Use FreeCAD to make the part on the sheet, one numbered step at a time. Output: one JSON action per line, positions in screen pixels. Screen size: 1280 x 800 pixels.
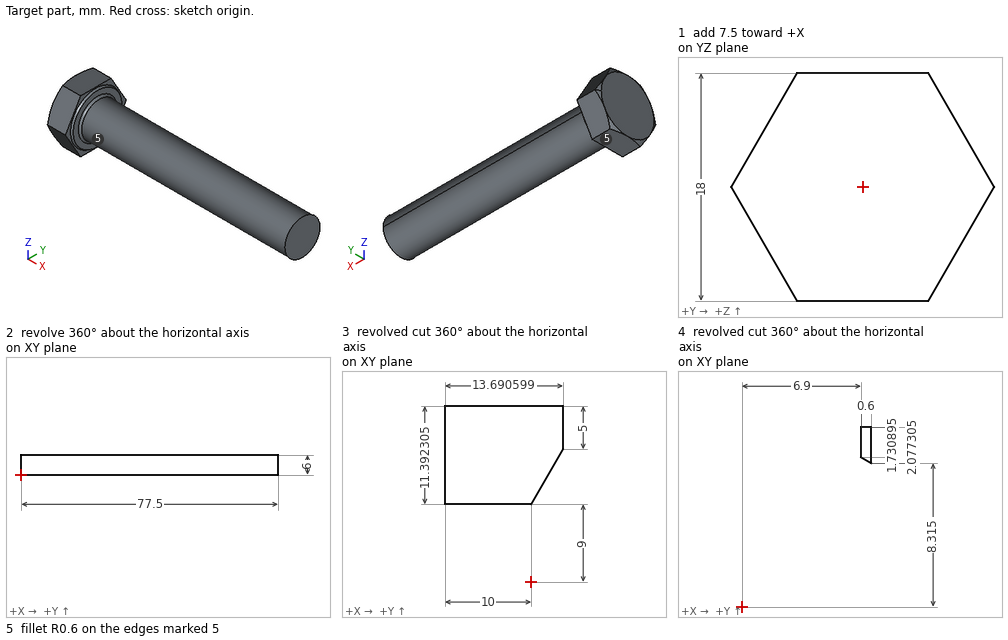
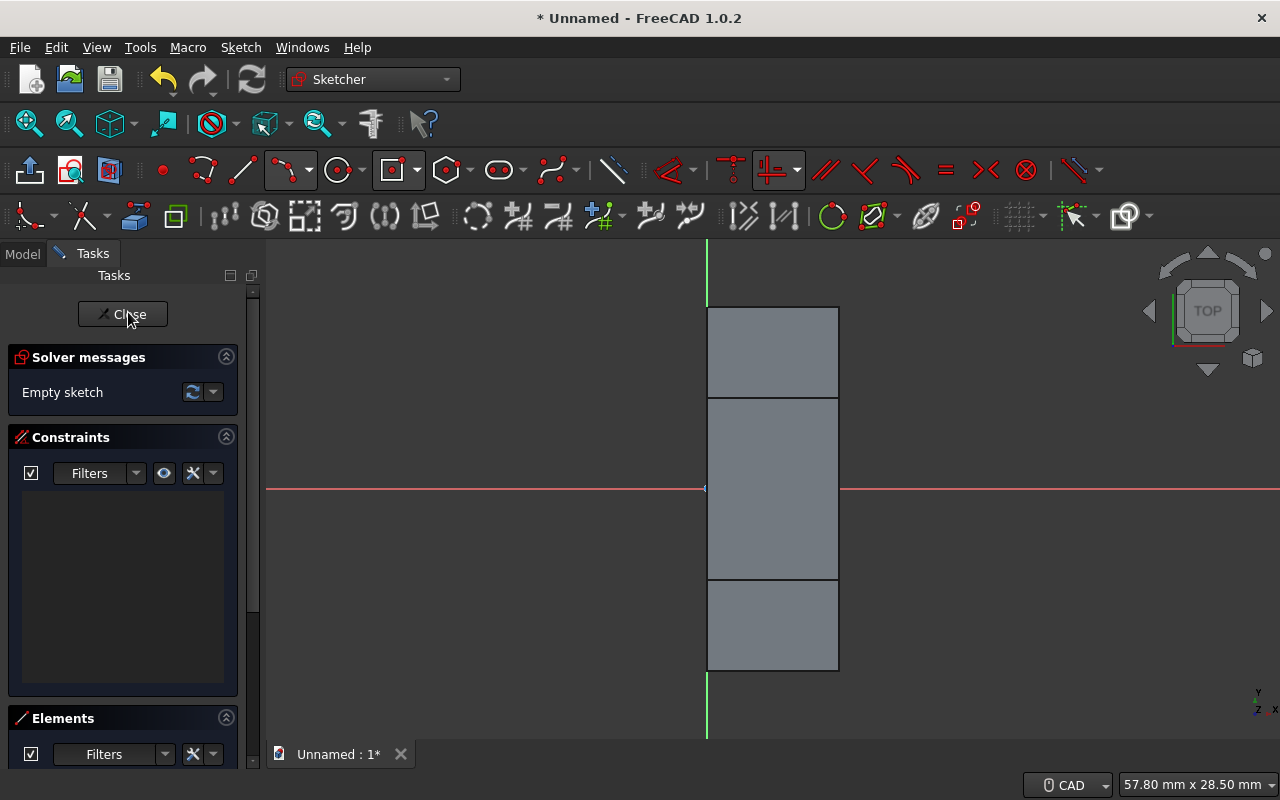
{"action": "left_click", "coordinate": [110, 170]}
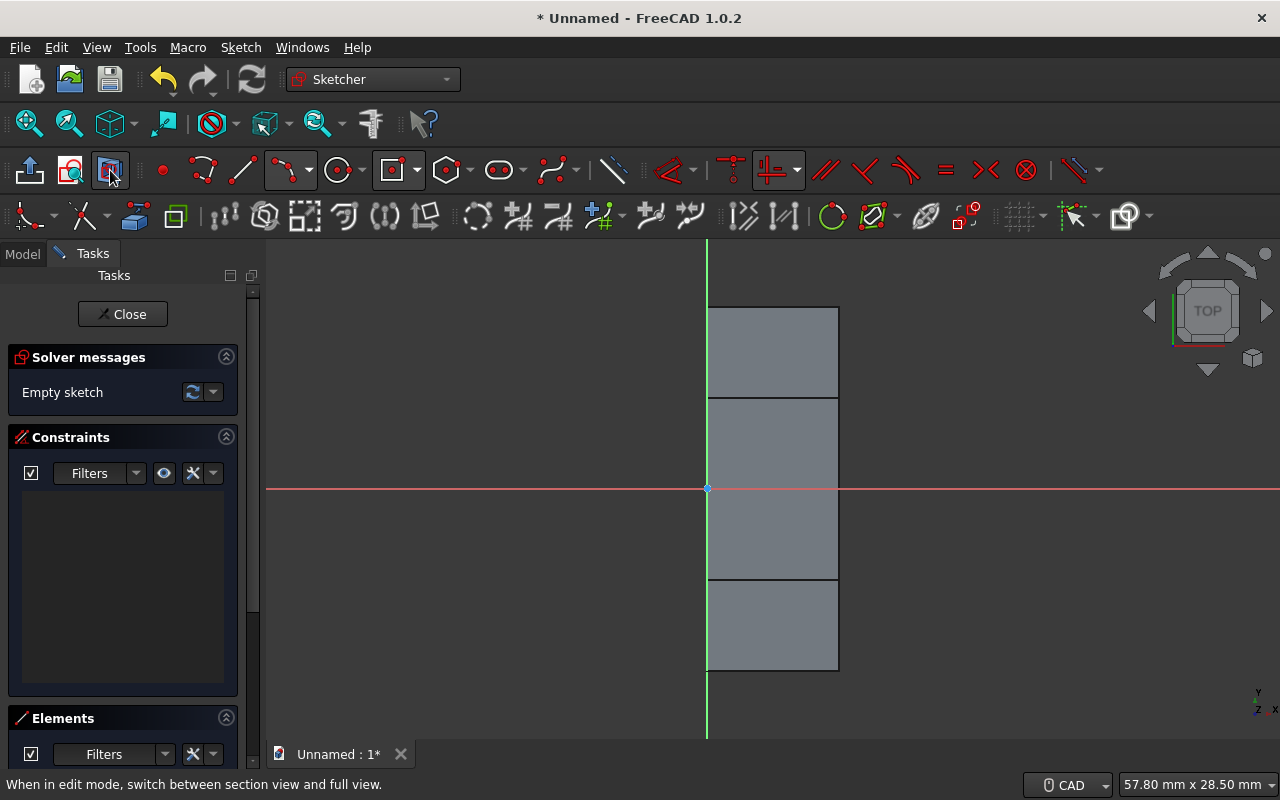
{"action": "scroll", "coordinate": [307, 520], "scroll_direction": "down", "scroll_amount": 5}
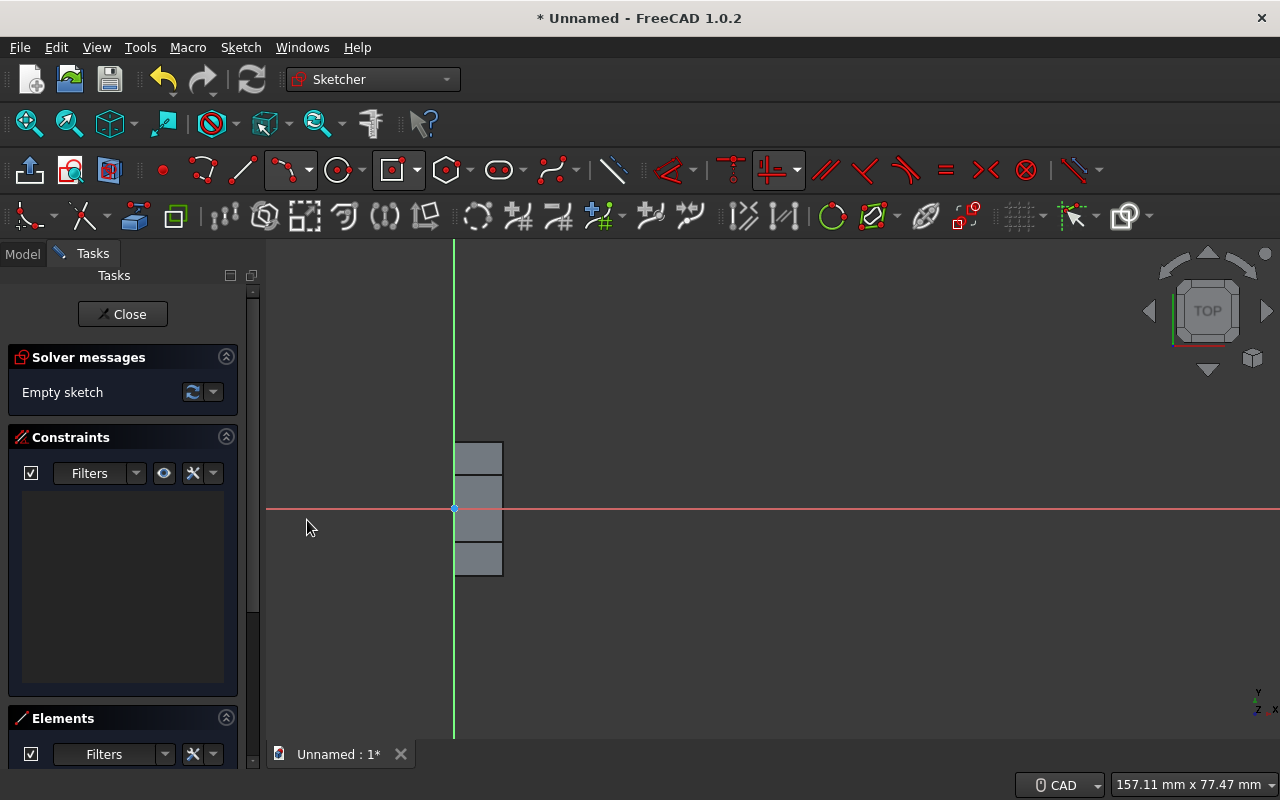
{"action": "key", "text": "g r"}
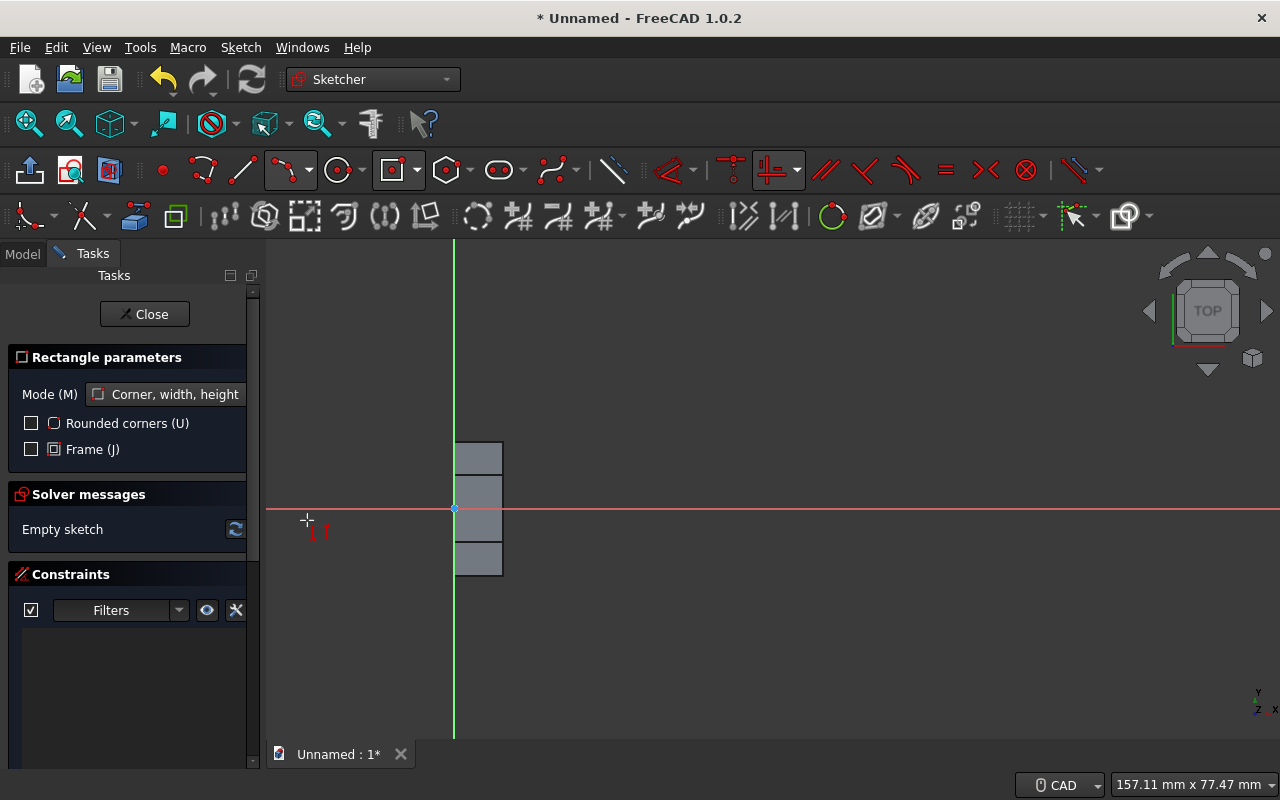
{"action": "left_click", "coordinate": [454, 509]}
{"action": "left_click", "coordinate": [954, 470]}
{"action": "key", "text": "Escape"}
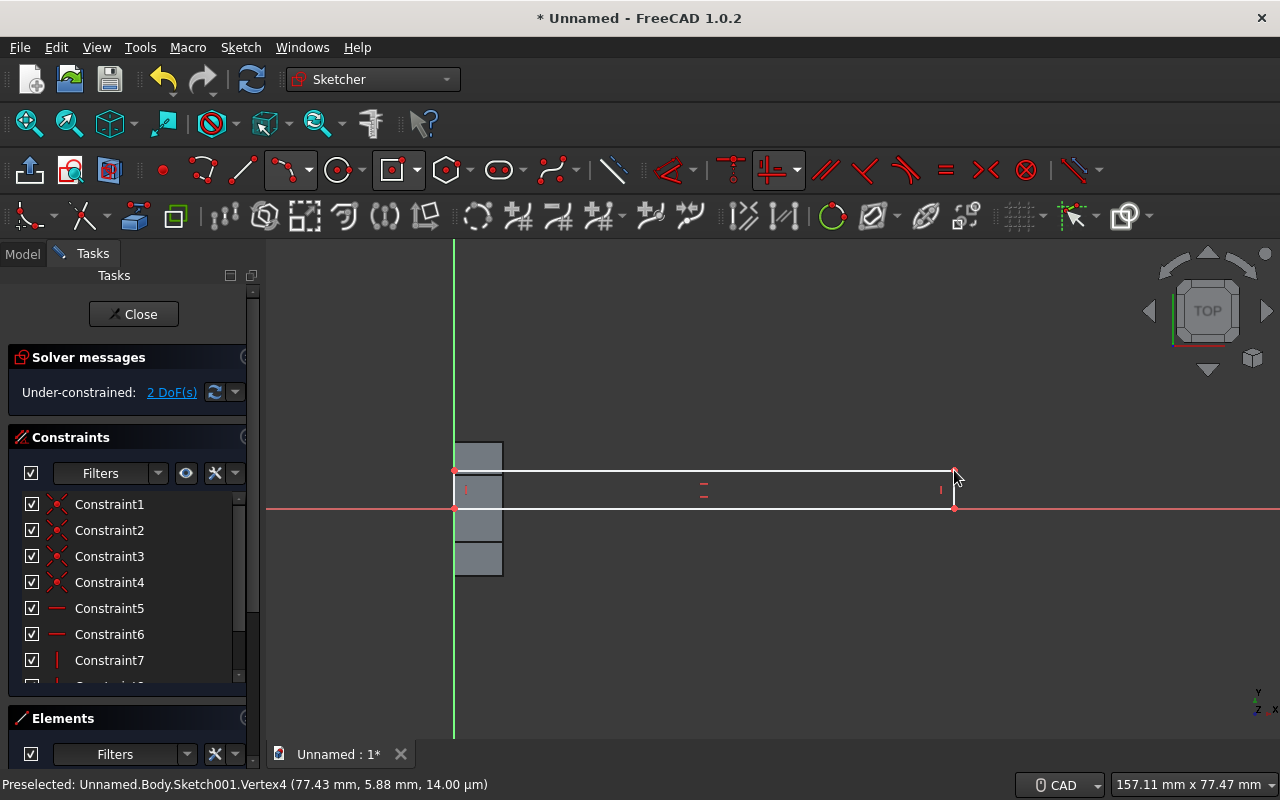
{"action": "left_click", "coordinate": [668, 170]}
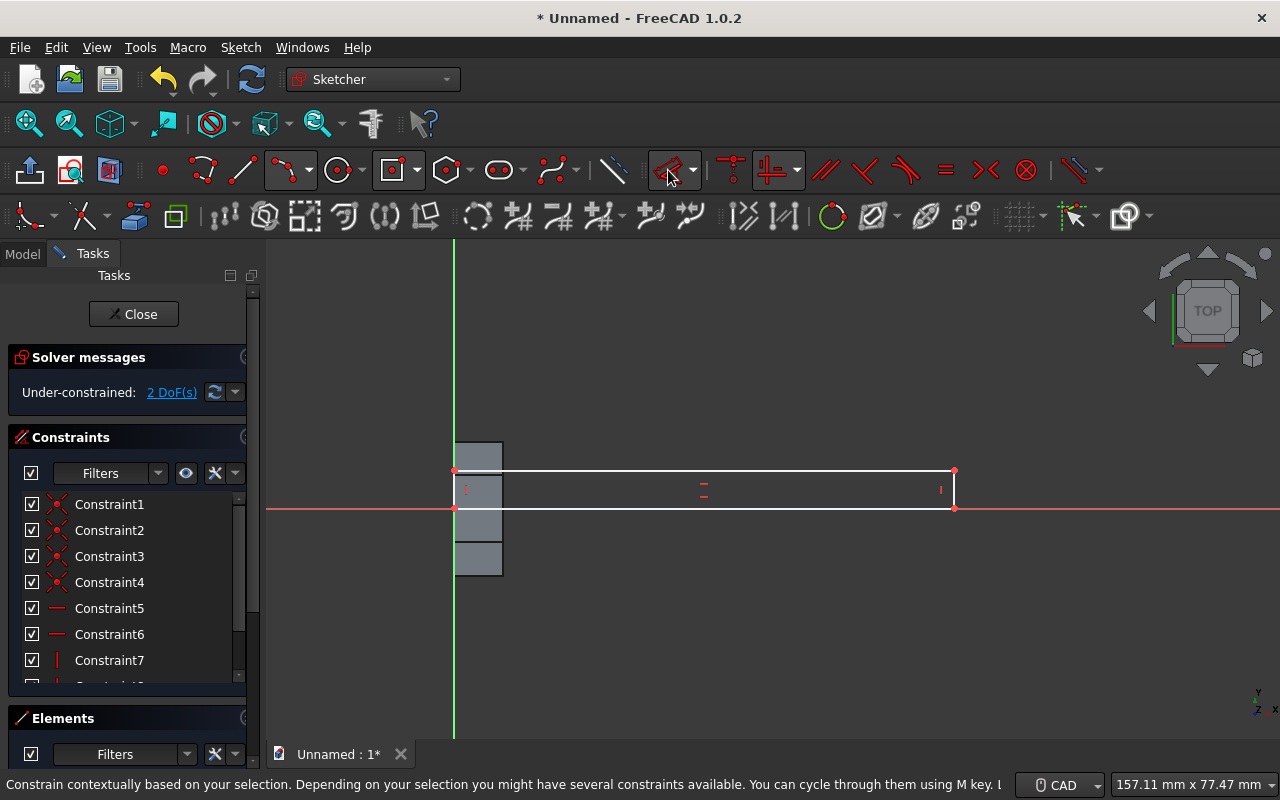
{"action": "left_click", "coordinate": [954, 498]}
{"action": "left_click", "coordinate": [988, 490]}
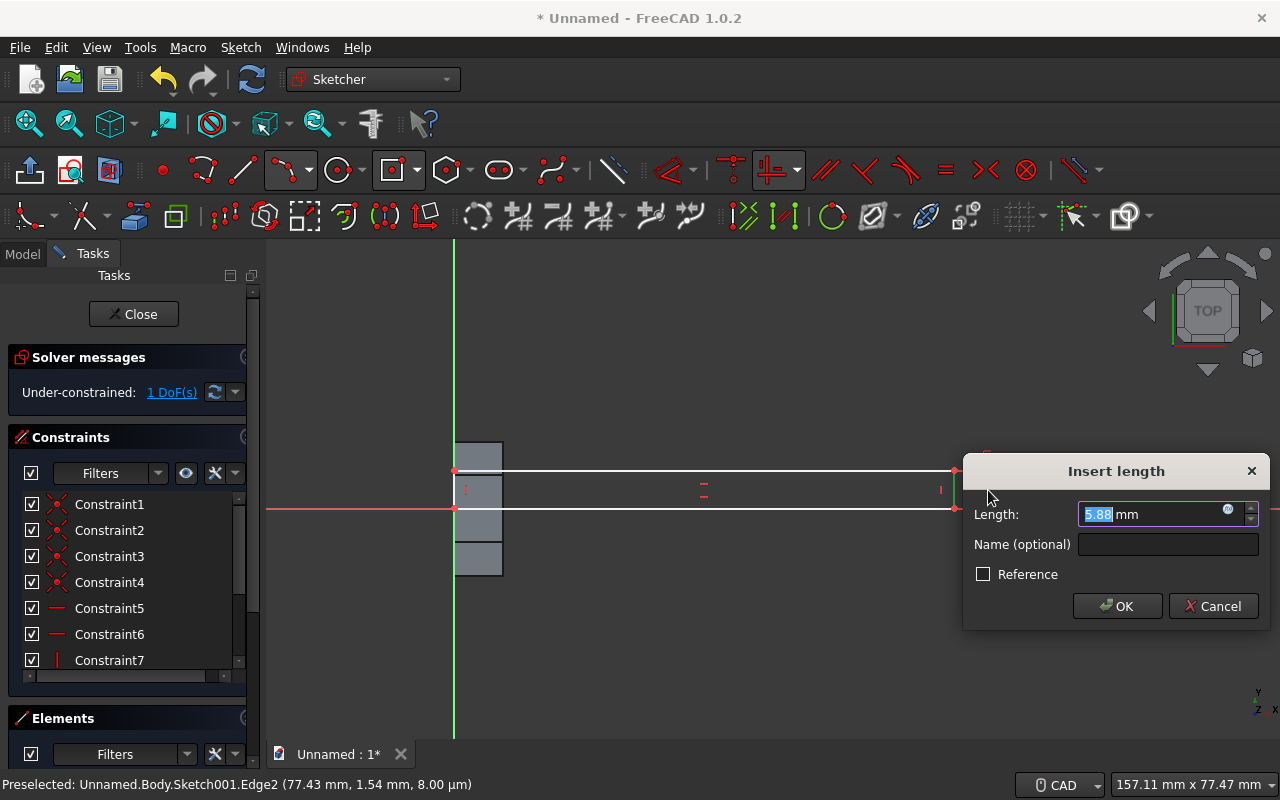
{"action": "type", "text": "6"}
{"action": "key", "text": "Return"}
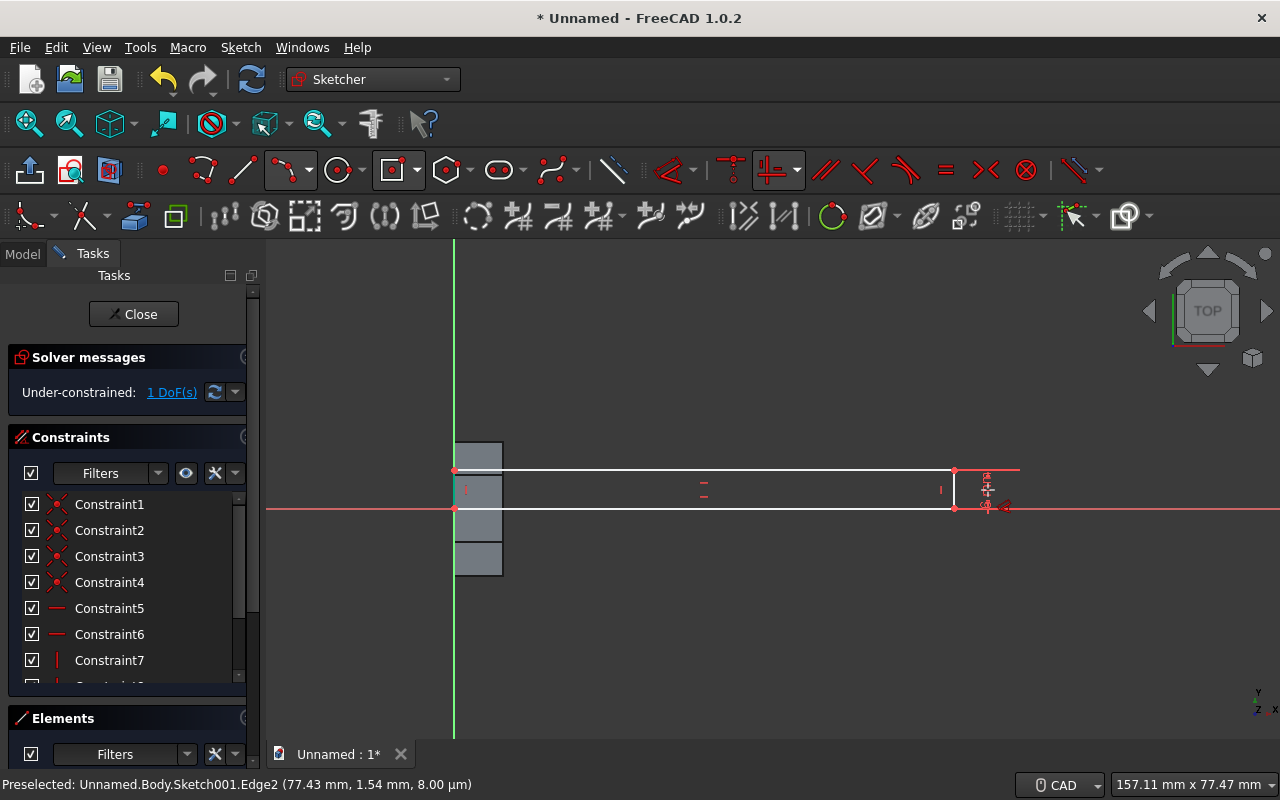
{"action": "left_click", "coordinate": [604, 509]}
{"action": "left_click", "coordinate": [704, 543]}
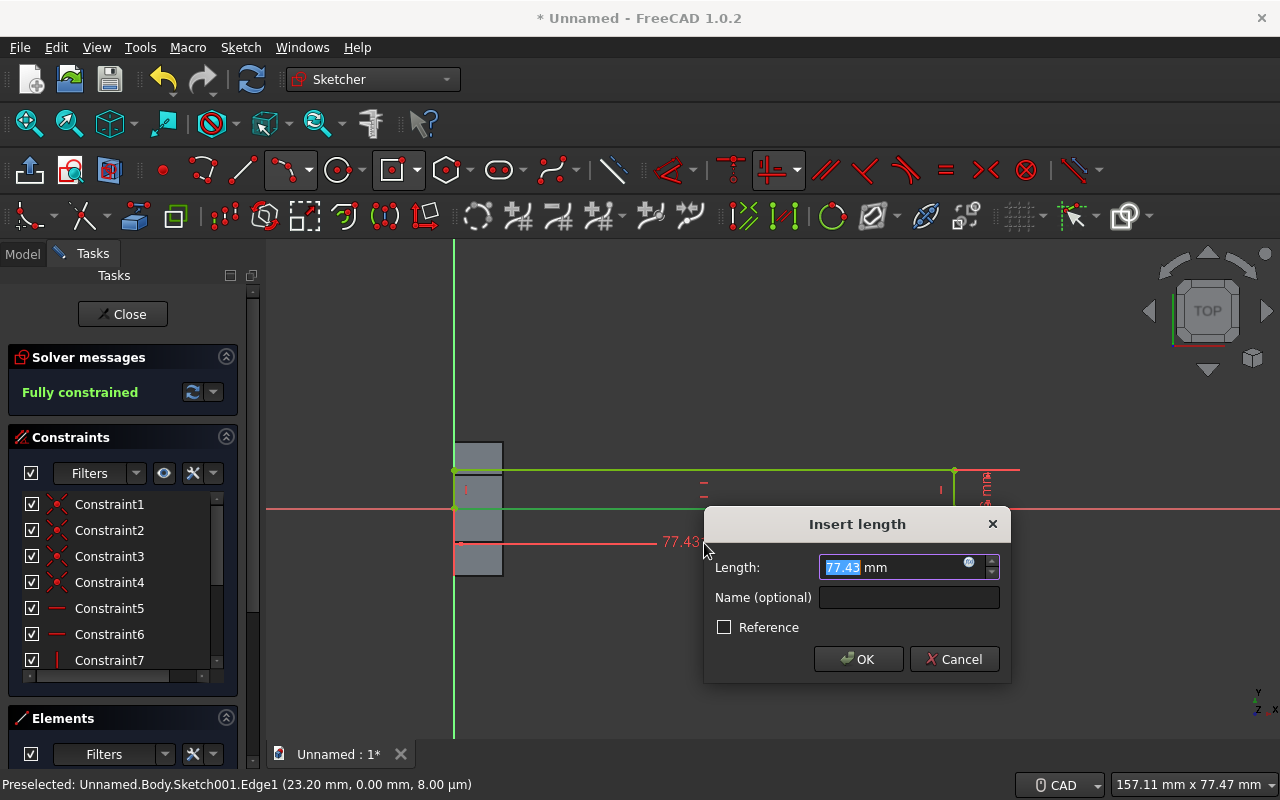
{"action": "type", "text": "77.5"}
{"action": "key", "text": "Return"}
{"action": "key", "text": "Escape"}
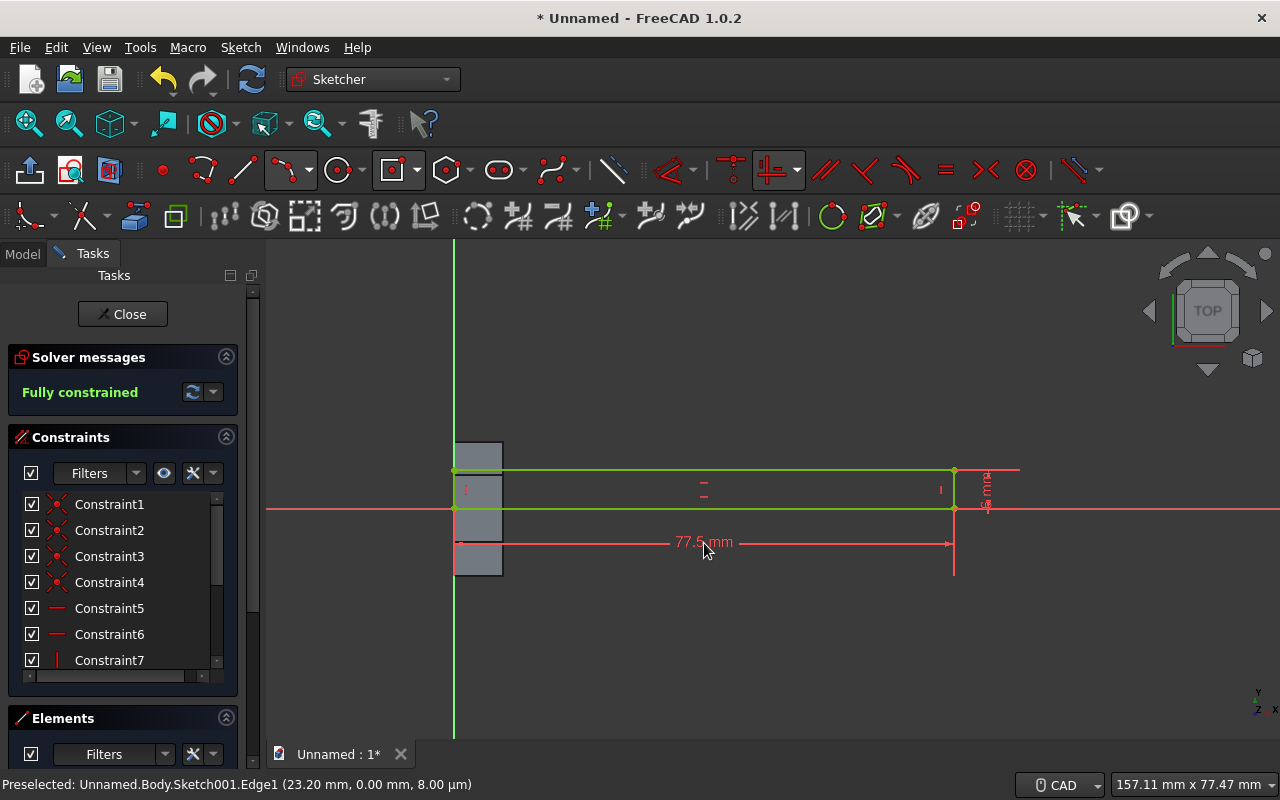
{"action": "left_click", "coordinate": [123, 314]}